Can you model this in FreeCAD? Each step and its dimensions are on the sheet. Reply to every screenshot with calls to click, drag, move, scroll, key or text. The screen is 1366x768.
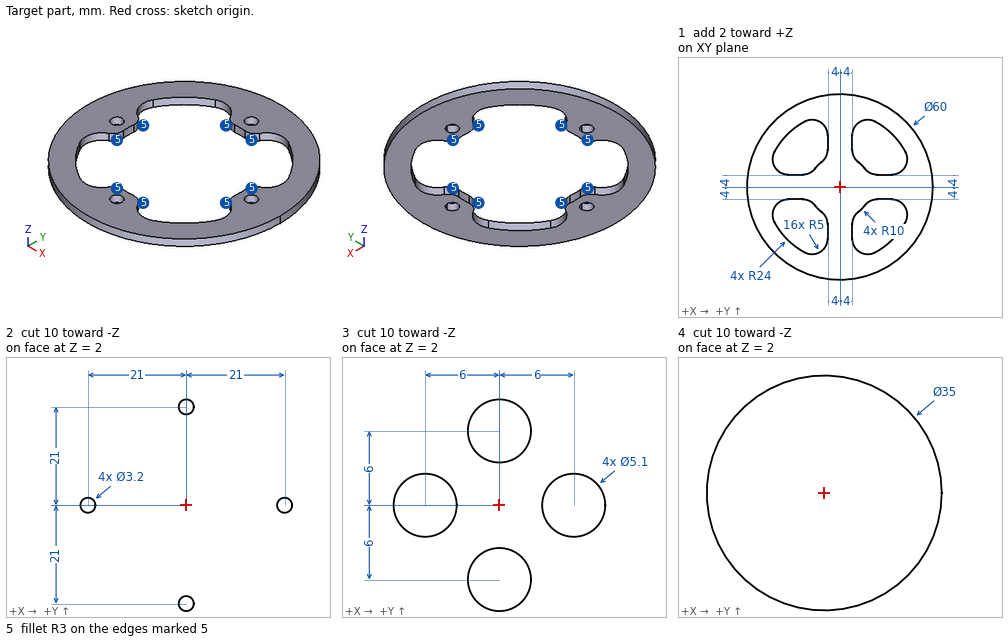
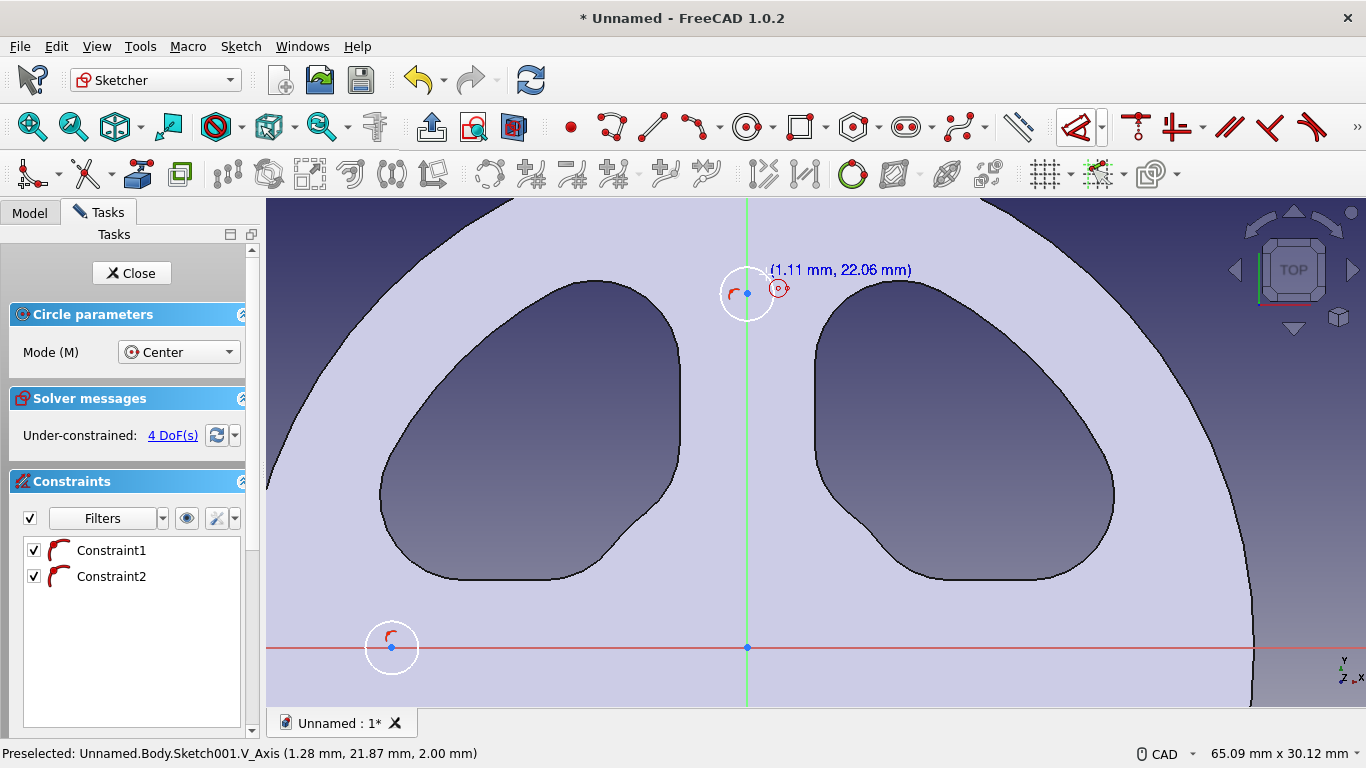
click(1102, 648)
click(1121, 629)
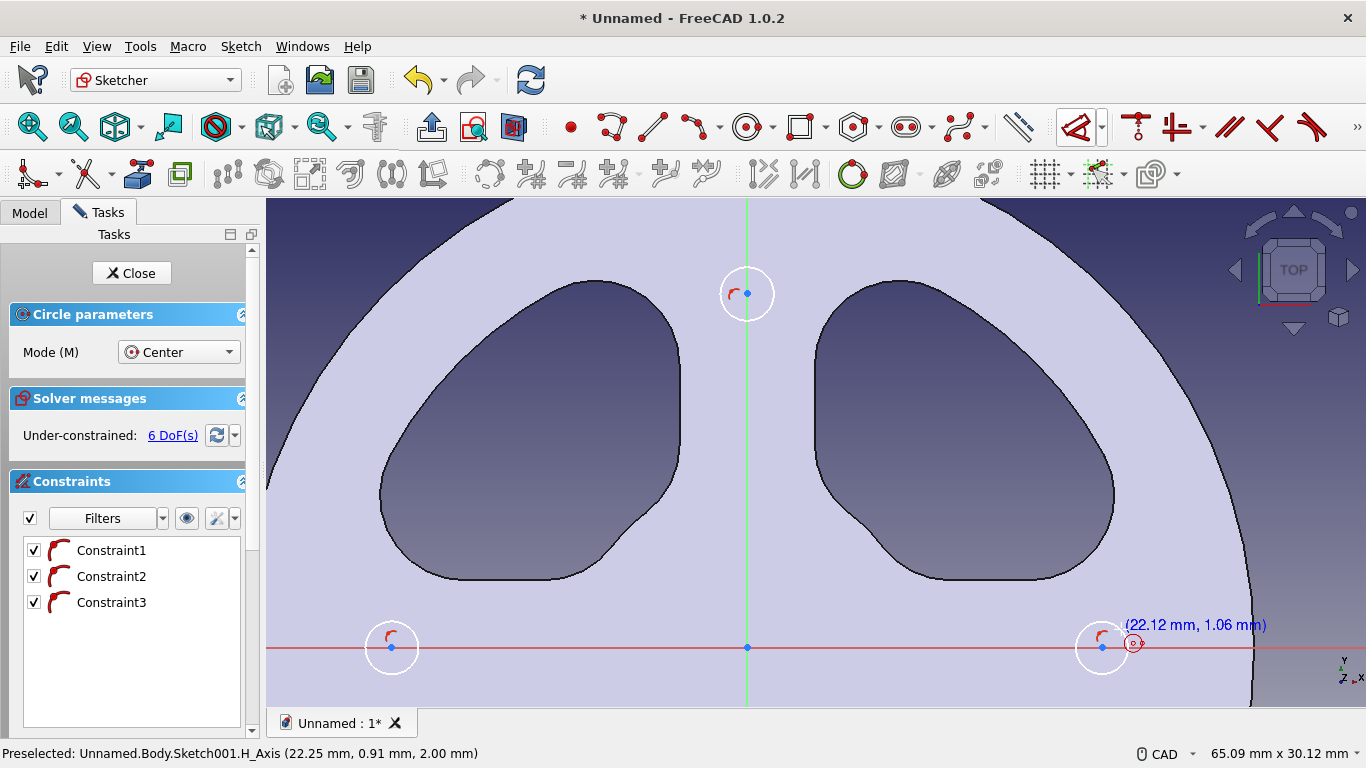
scroll(748, 293, down, 4)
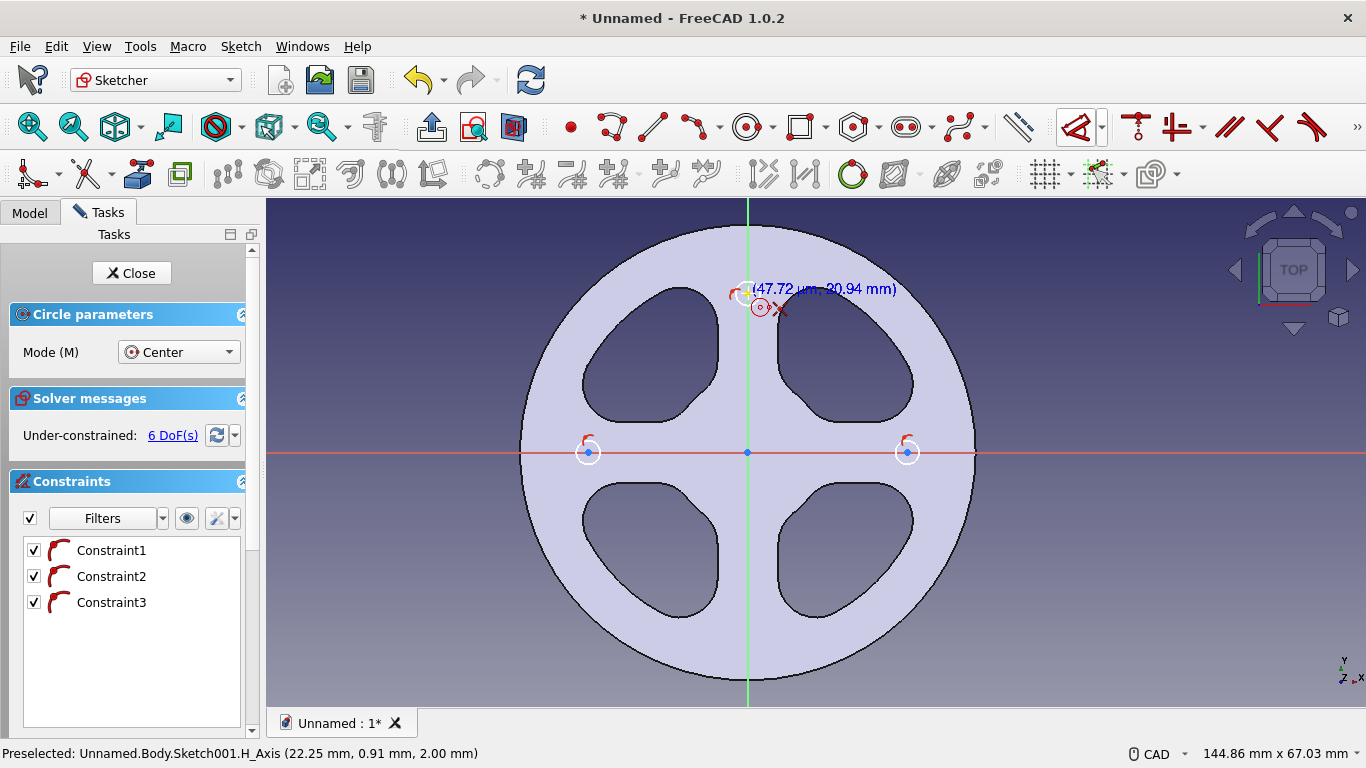
scroll(748, 612, up, 4)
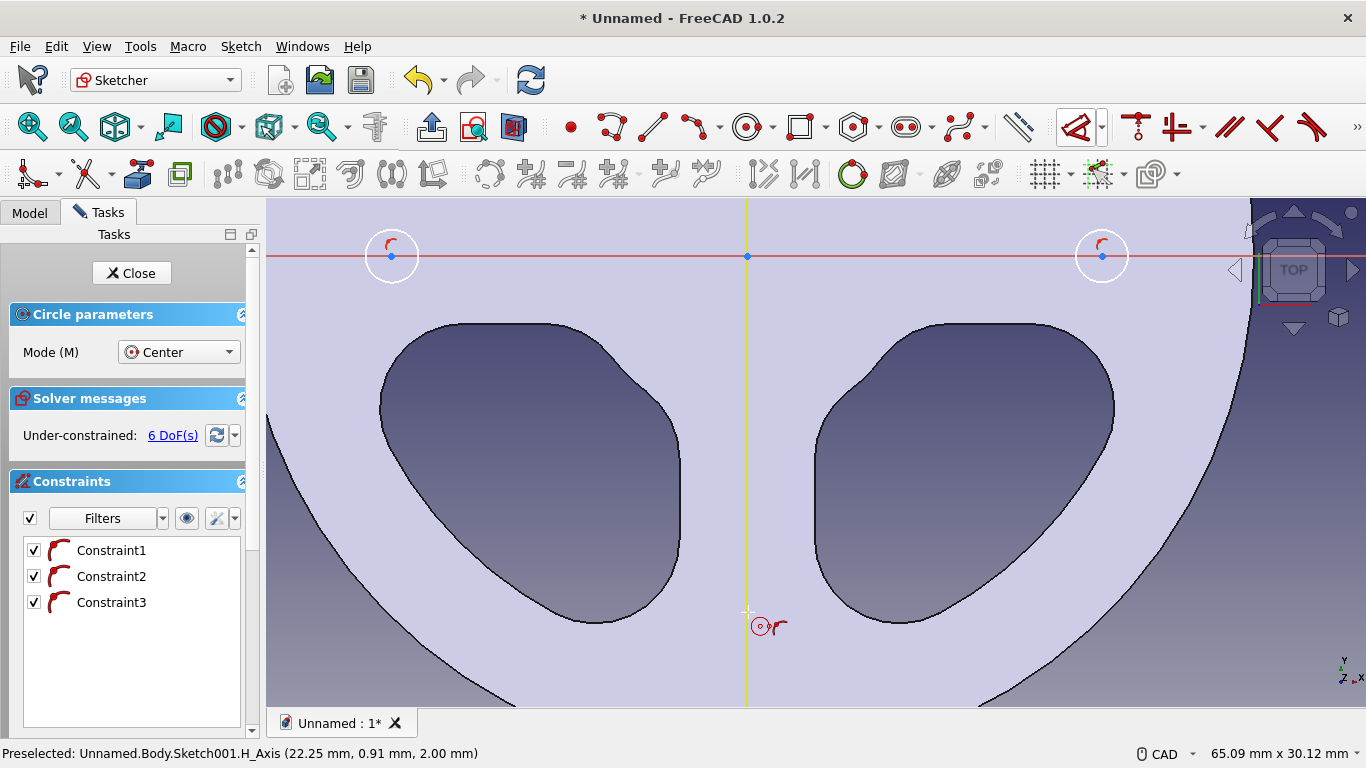
click(747, 611)
click(766, 592)
key(Escape)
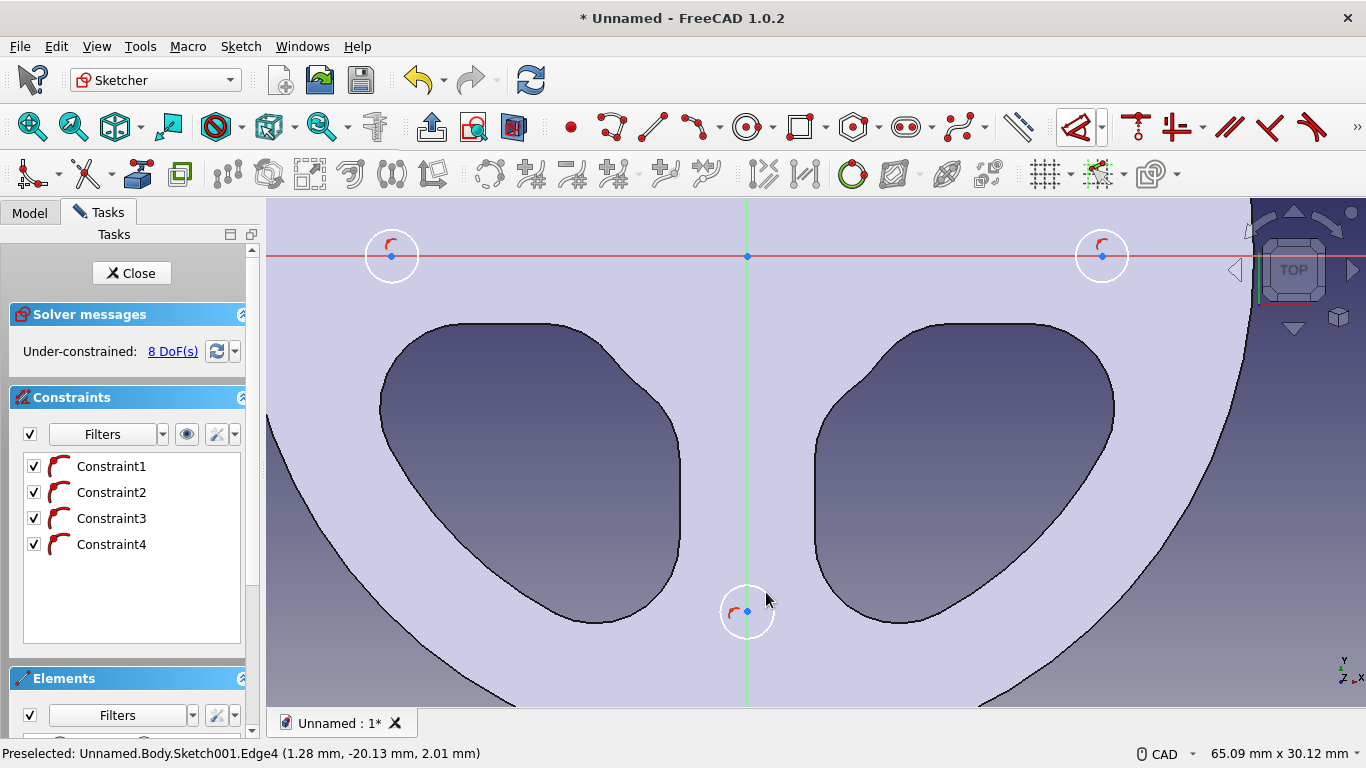
click(411, 237)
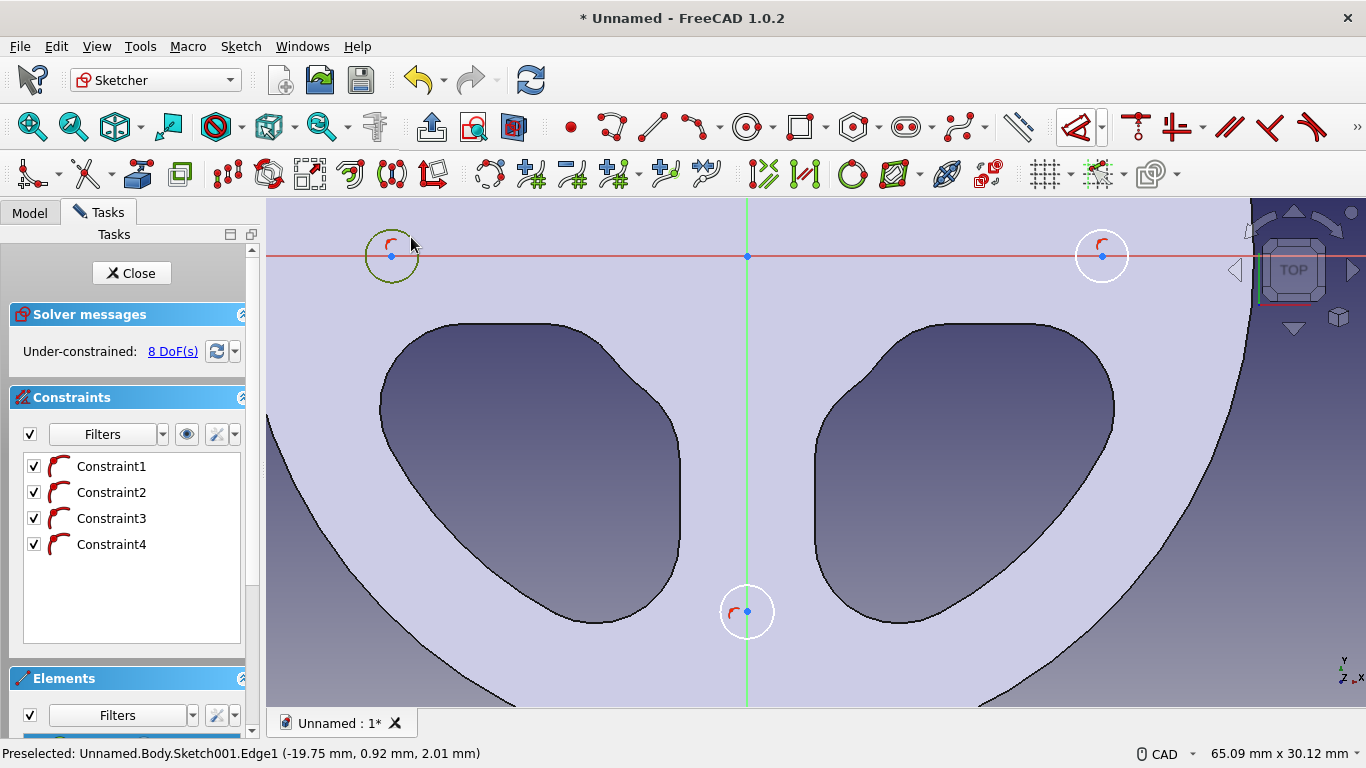
scroll(748, 613, down, 4)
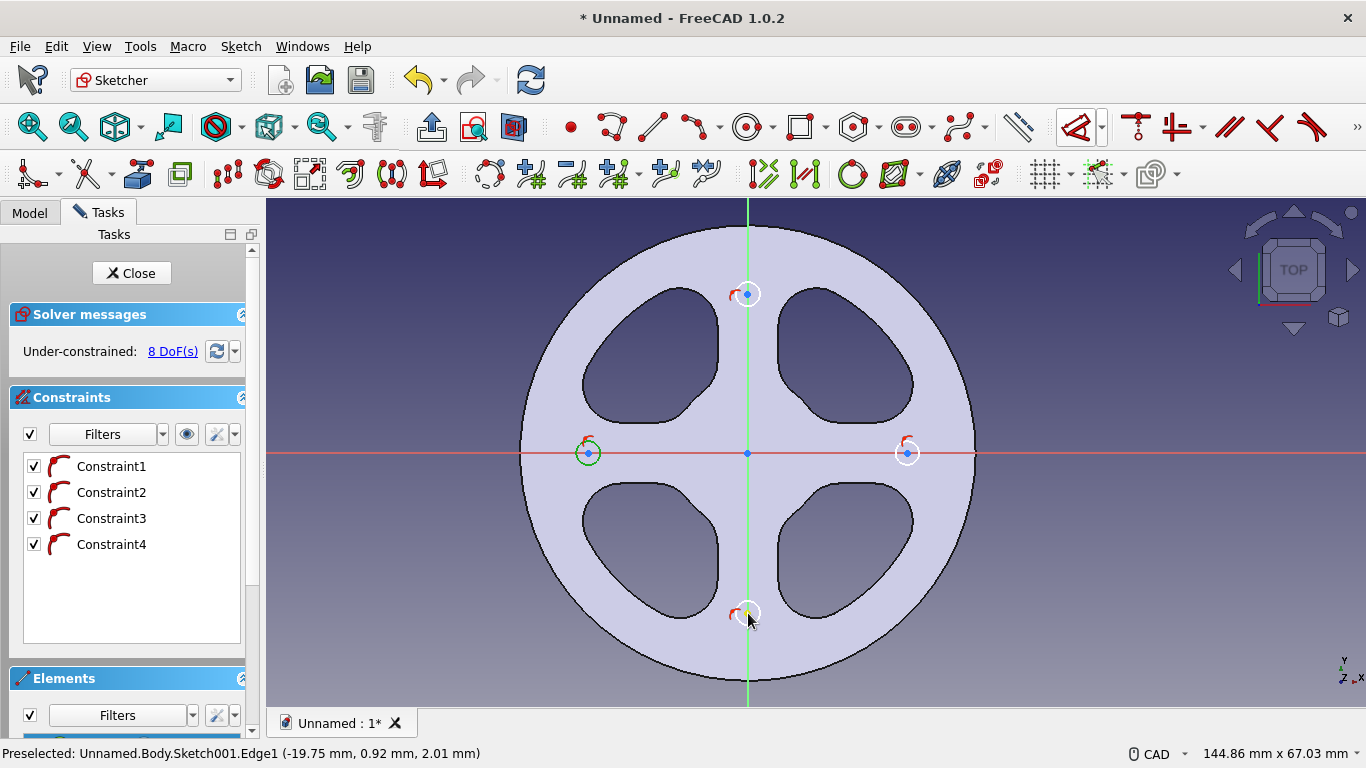
scroll(756, 286, up, 3)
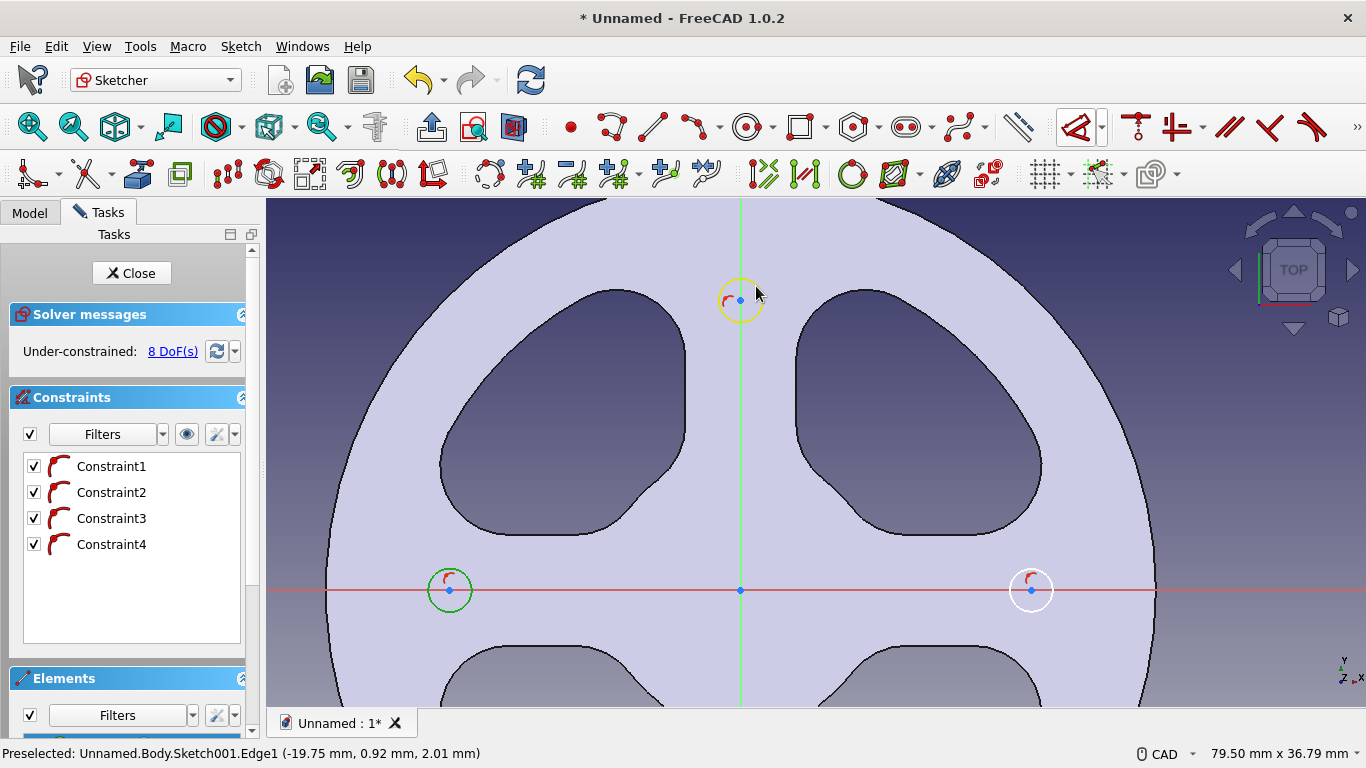
click(756, 285)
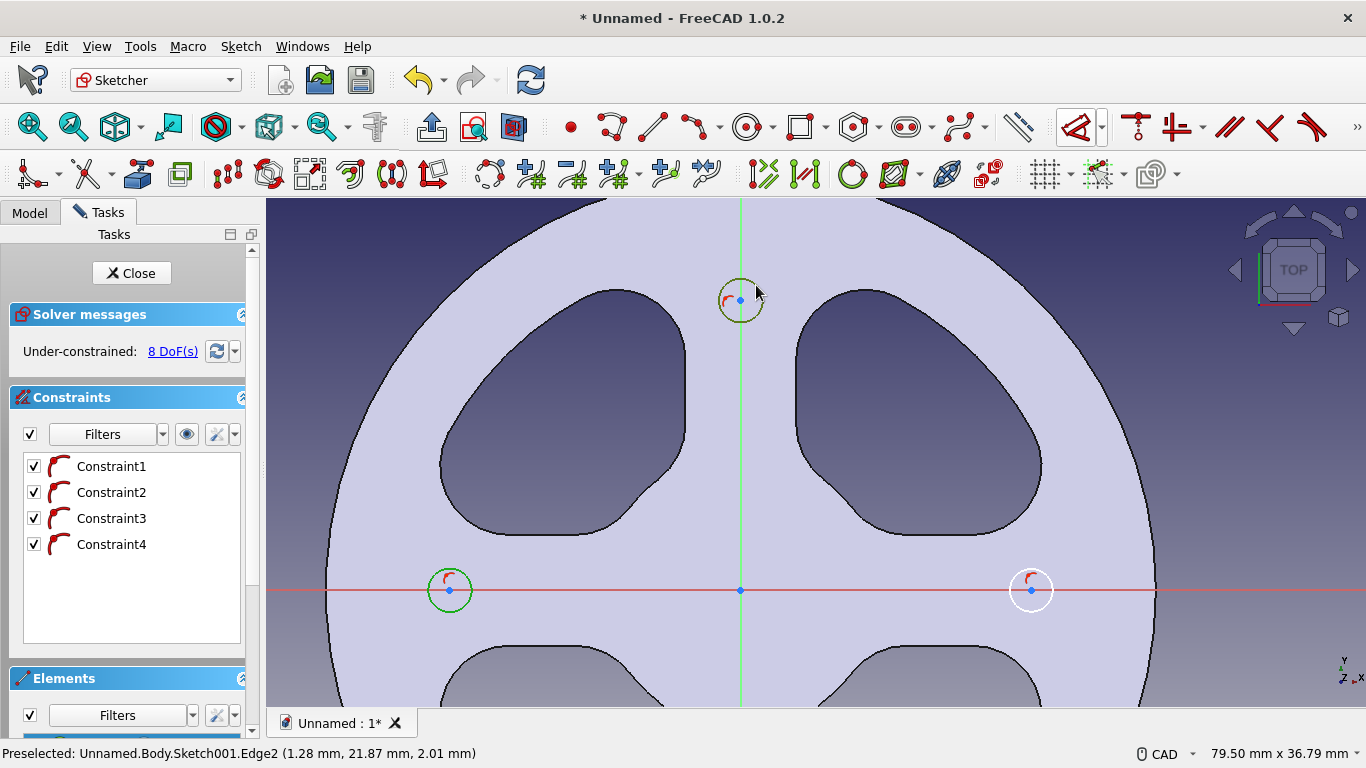
click(1046, 575)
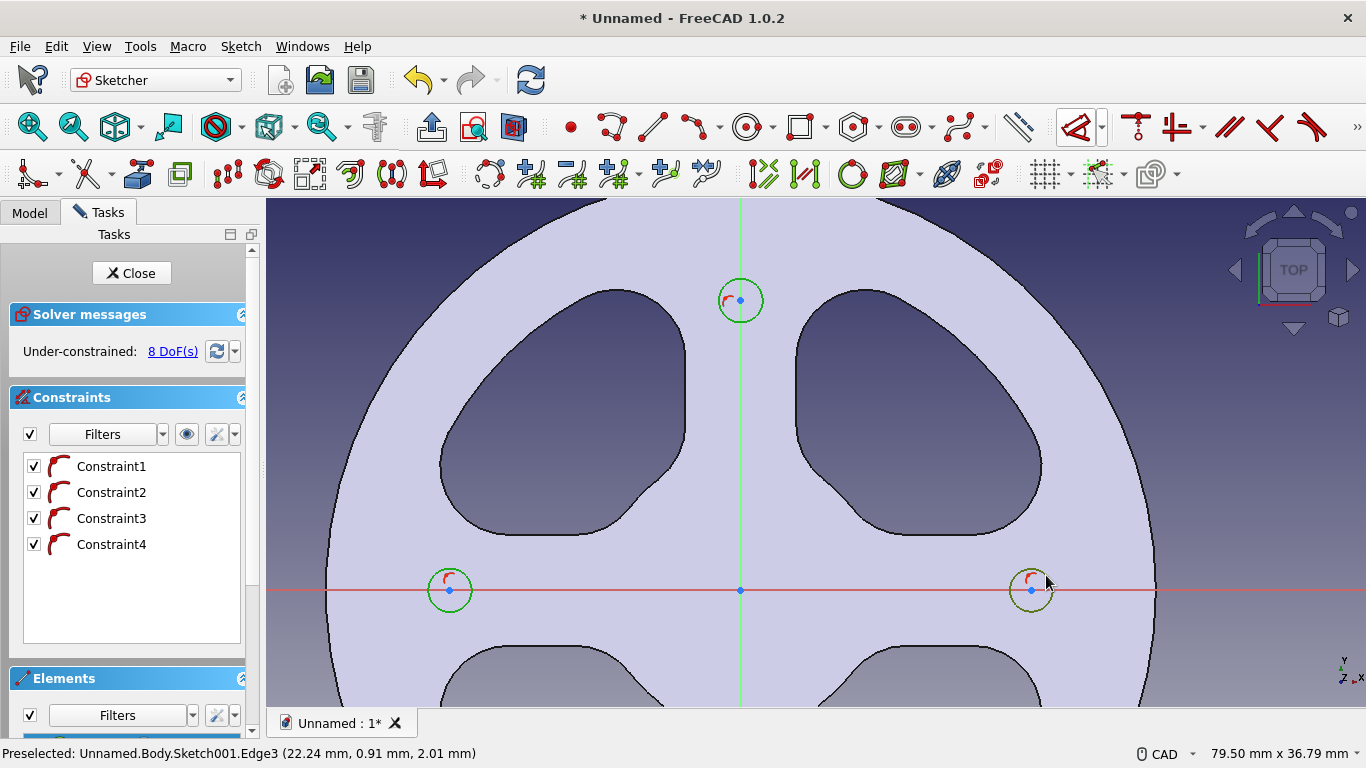
scroll(756, 285, down, 3)